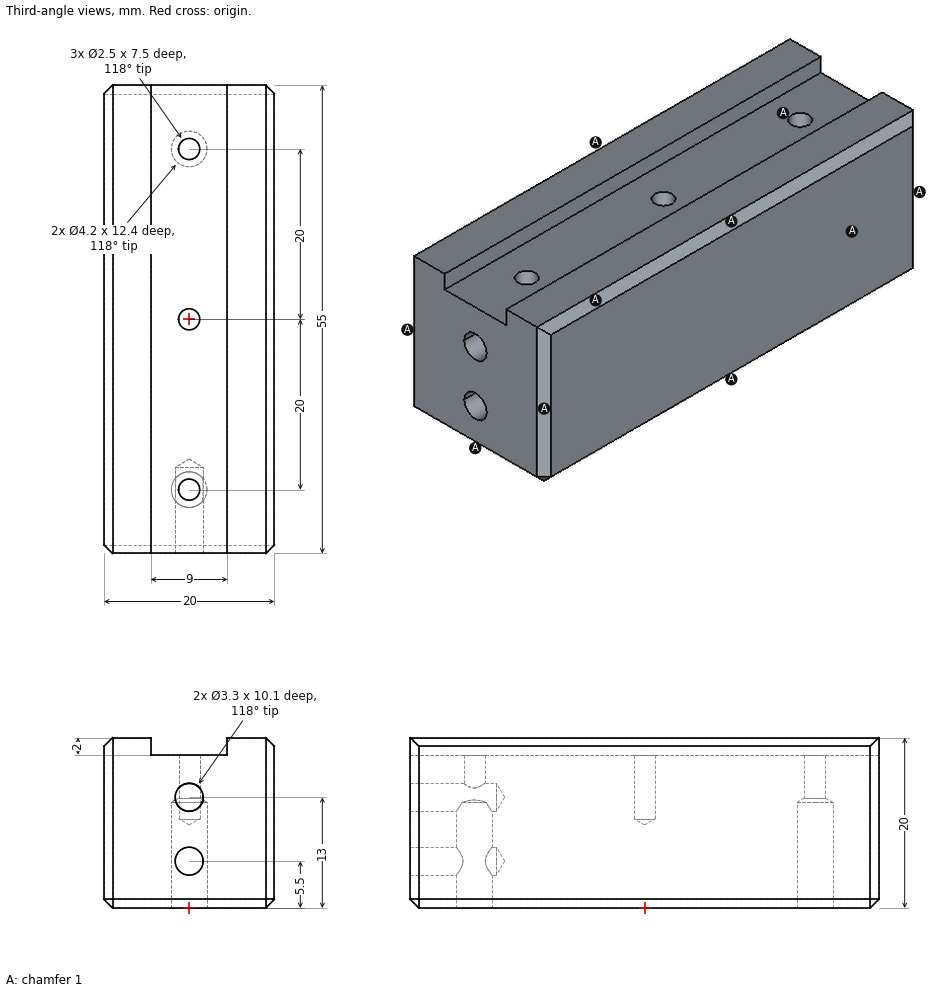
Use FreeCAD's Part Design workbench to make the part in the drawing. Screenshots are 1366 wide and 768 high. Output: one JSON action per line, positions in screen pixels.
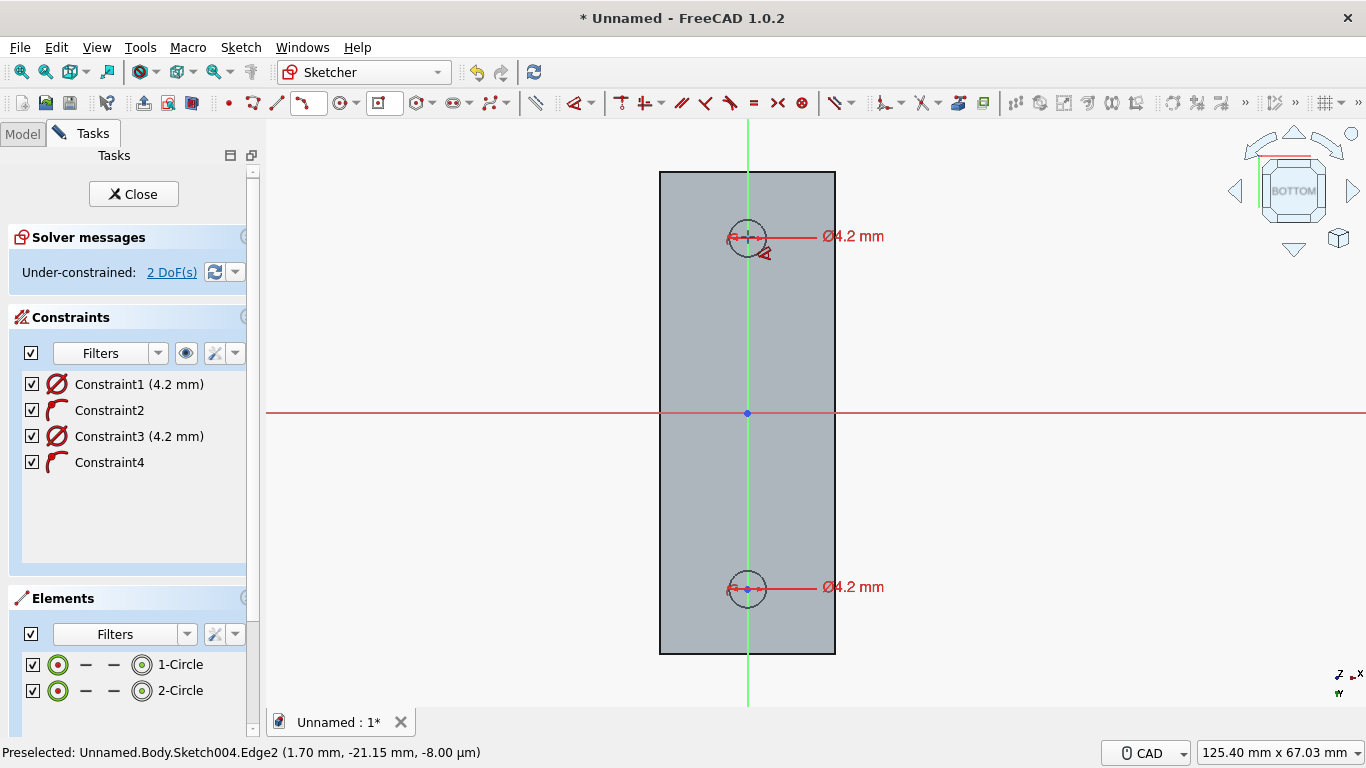
{"action": "left_click", "coordinate": [748, 589]}
{"action": "left_click", "coordinate": [782, 501]}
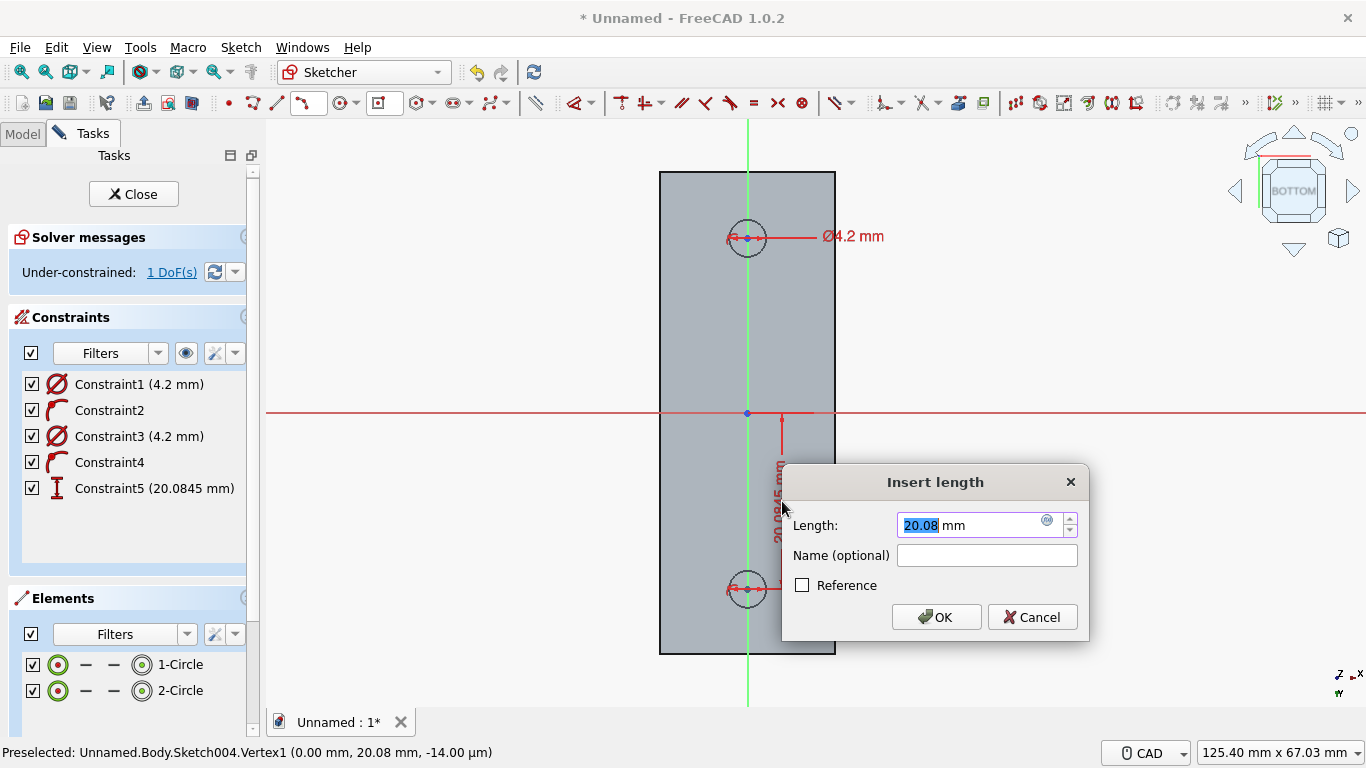
{"action": "type", "text": "20"}
{"action": "key", "text": "Return"}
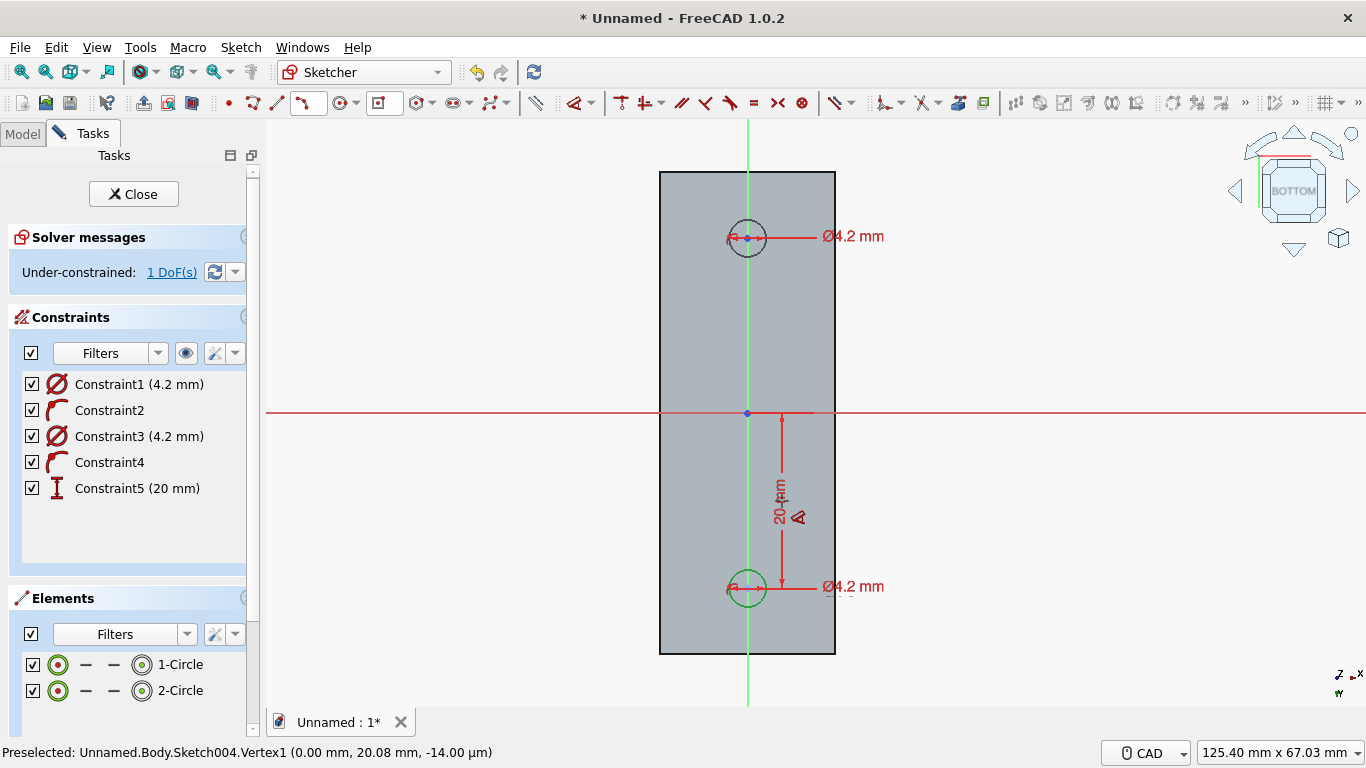
{"action": "left_click", "coordinate": [748, 238]}
{"action": "left_click", "coordinate": [782, 326]}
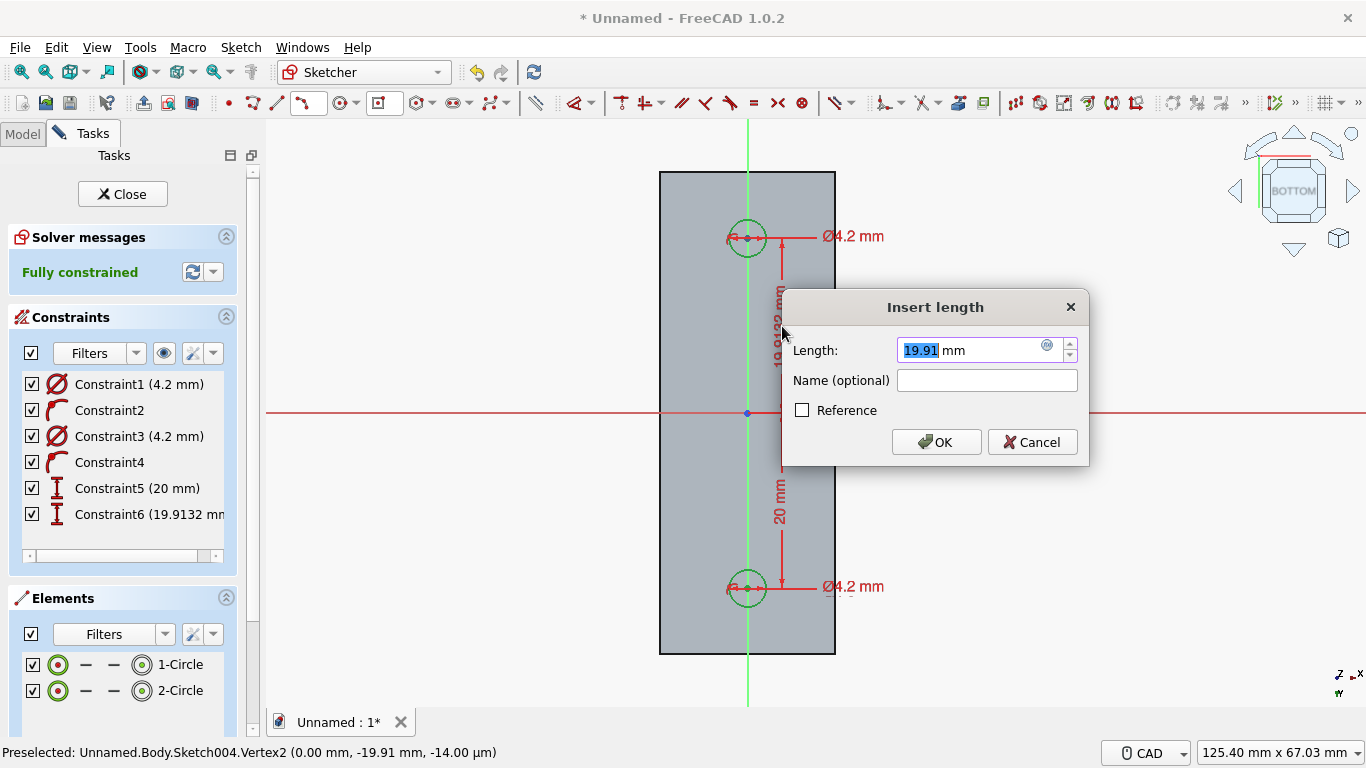
{"action": "type", "text": "20"}
{"action": "key", "text": "Return"}
{"action": "key", "text": "Escape"}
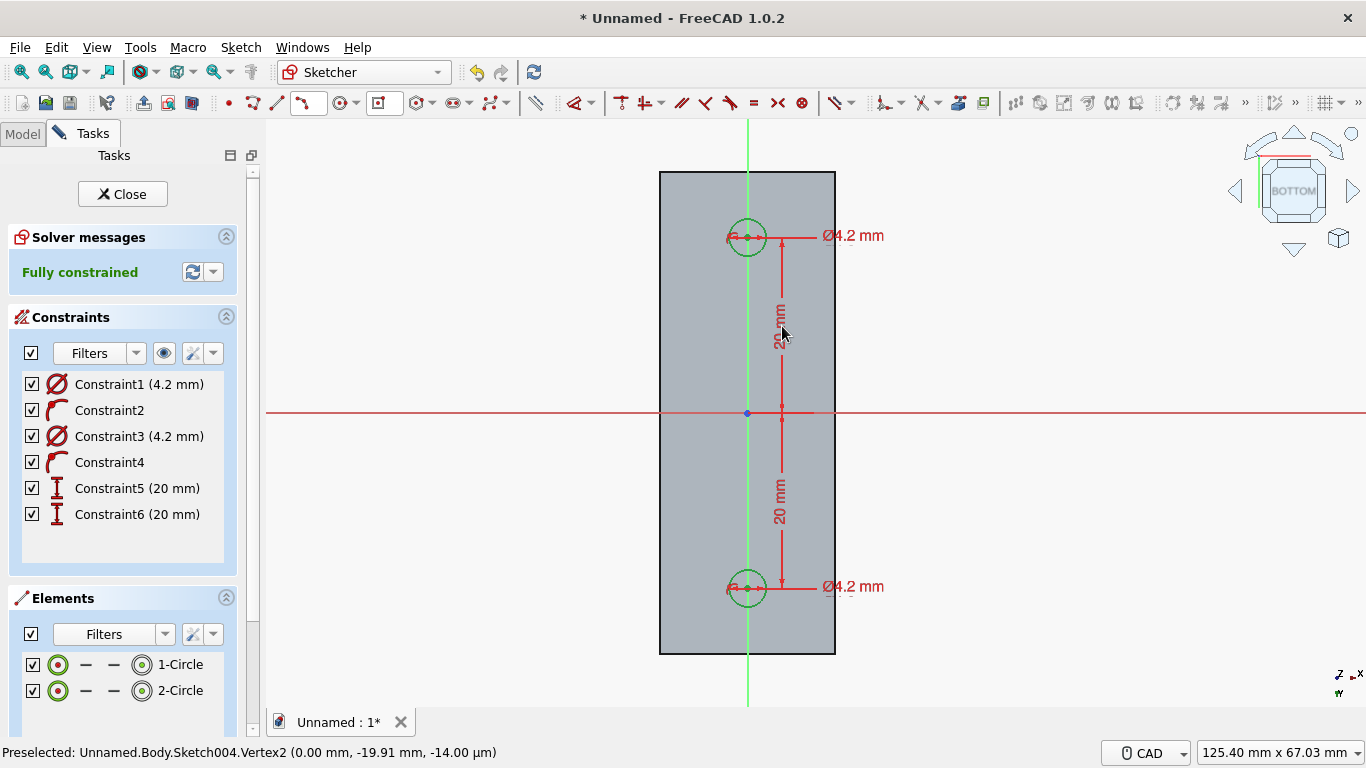
{"action": "left_click", "coordinate": [123, 194]}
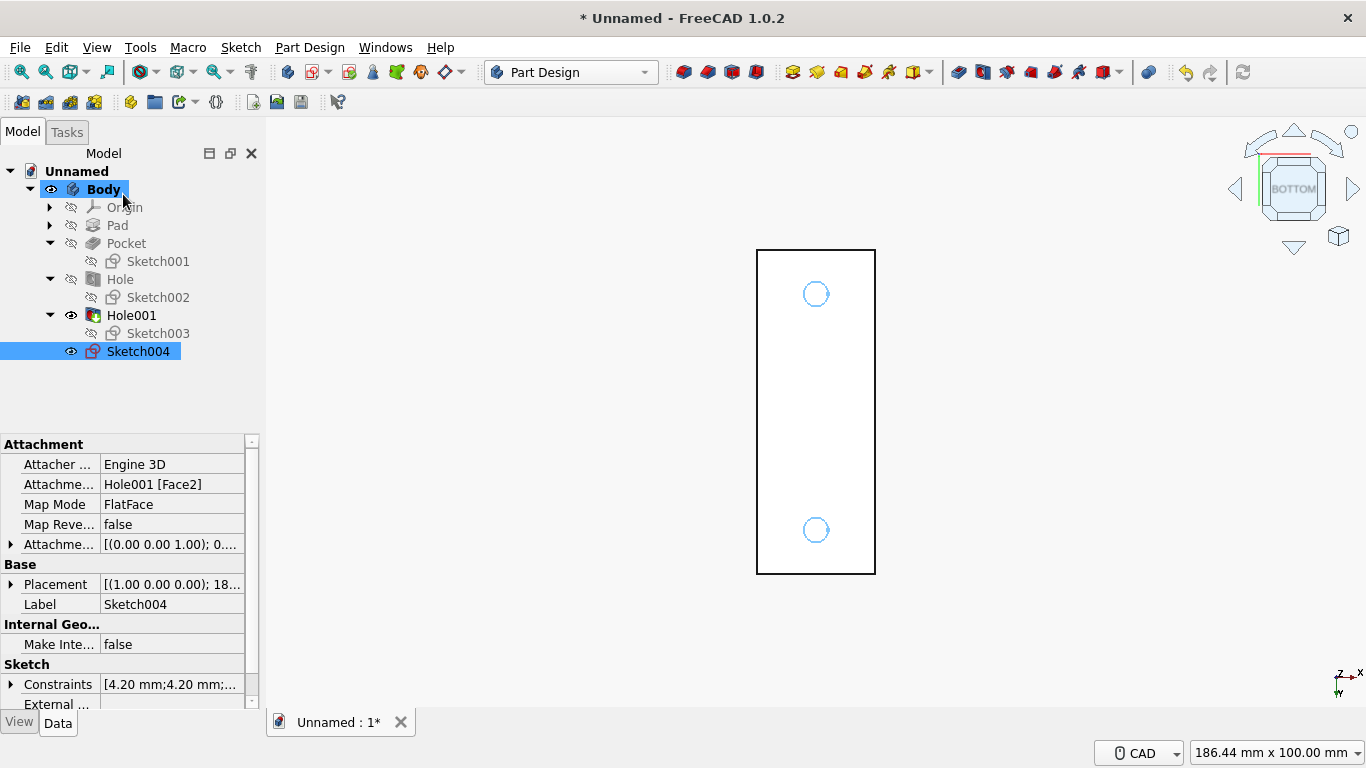
{"action": "left_click", "coordinate": [984, 72]}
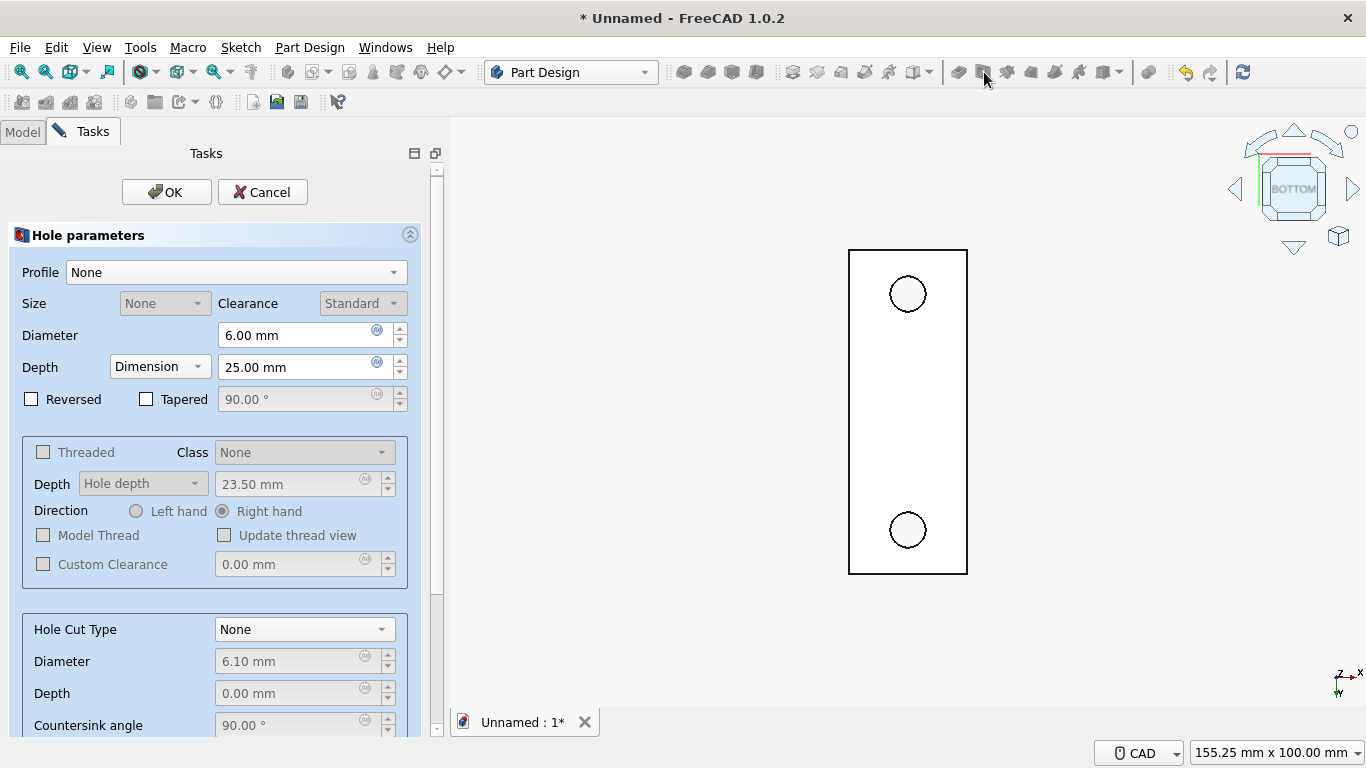
{"action": "triple_click", "coordinate": [305, 335]}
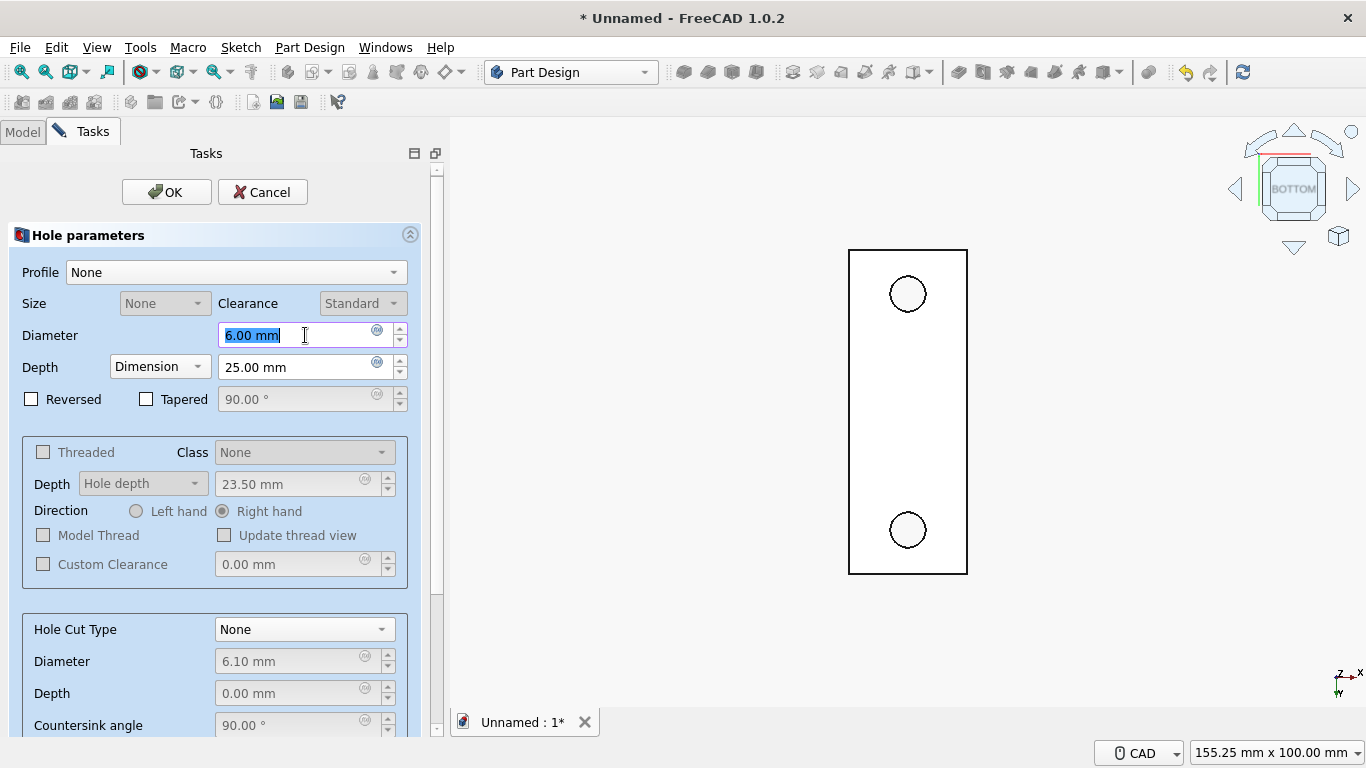
{"action": "type", "text": "4.2"}
{"action": "key", "text": "Tab"}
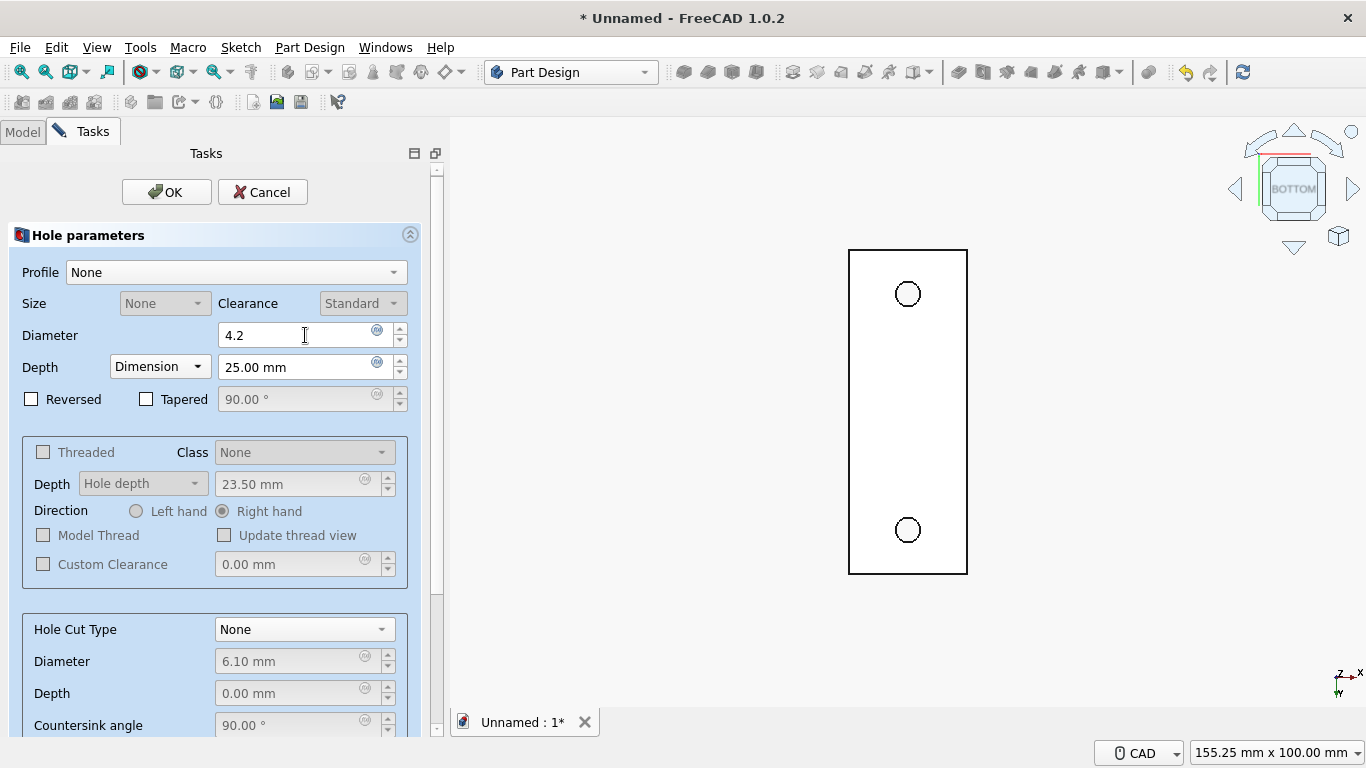
{"action": "triple_click", "coordinate": [305, 367]}